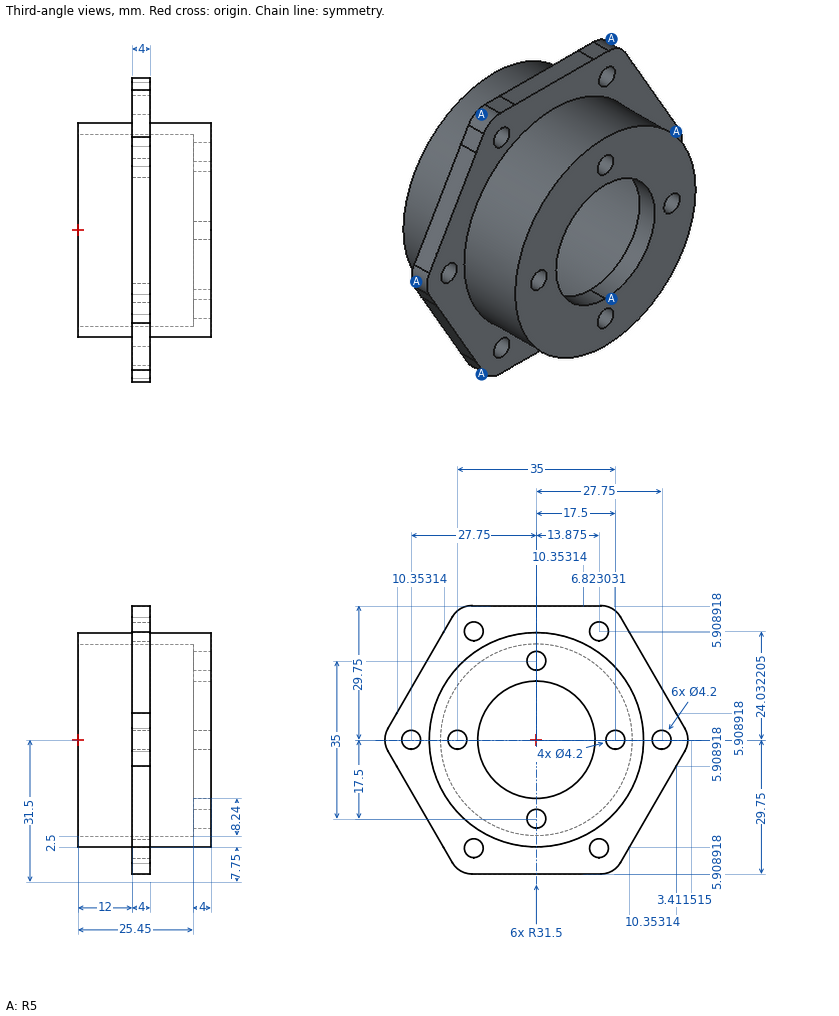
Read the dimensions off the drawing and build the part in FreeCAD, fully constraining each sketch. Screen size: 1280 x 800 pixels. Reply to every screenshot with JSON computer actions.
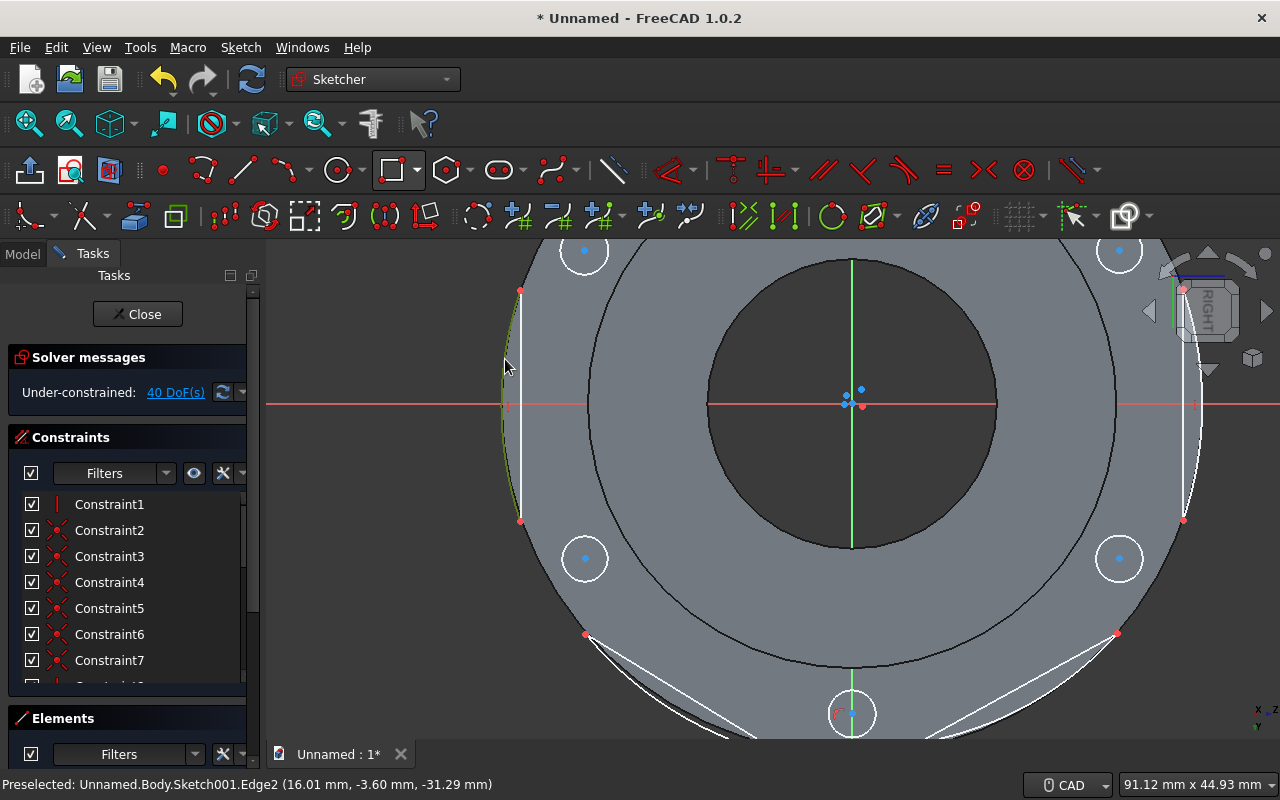
{"action": "scroll", "coordinate": [584, 558], "scroll_direction": "down", "scroll_amount": 4}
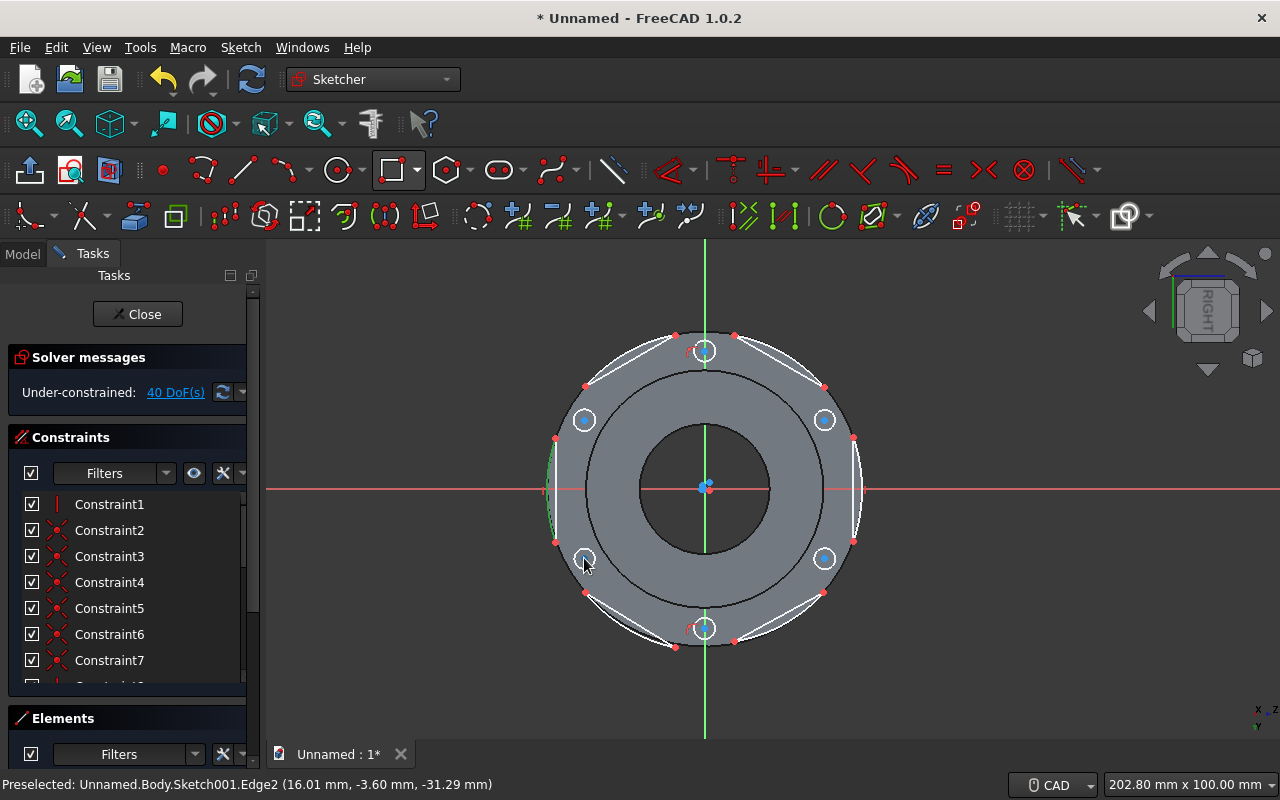
{"action": "scroll", "coordinate": [861, 511], "scroll_direction": "up", "scroll_amount": 4}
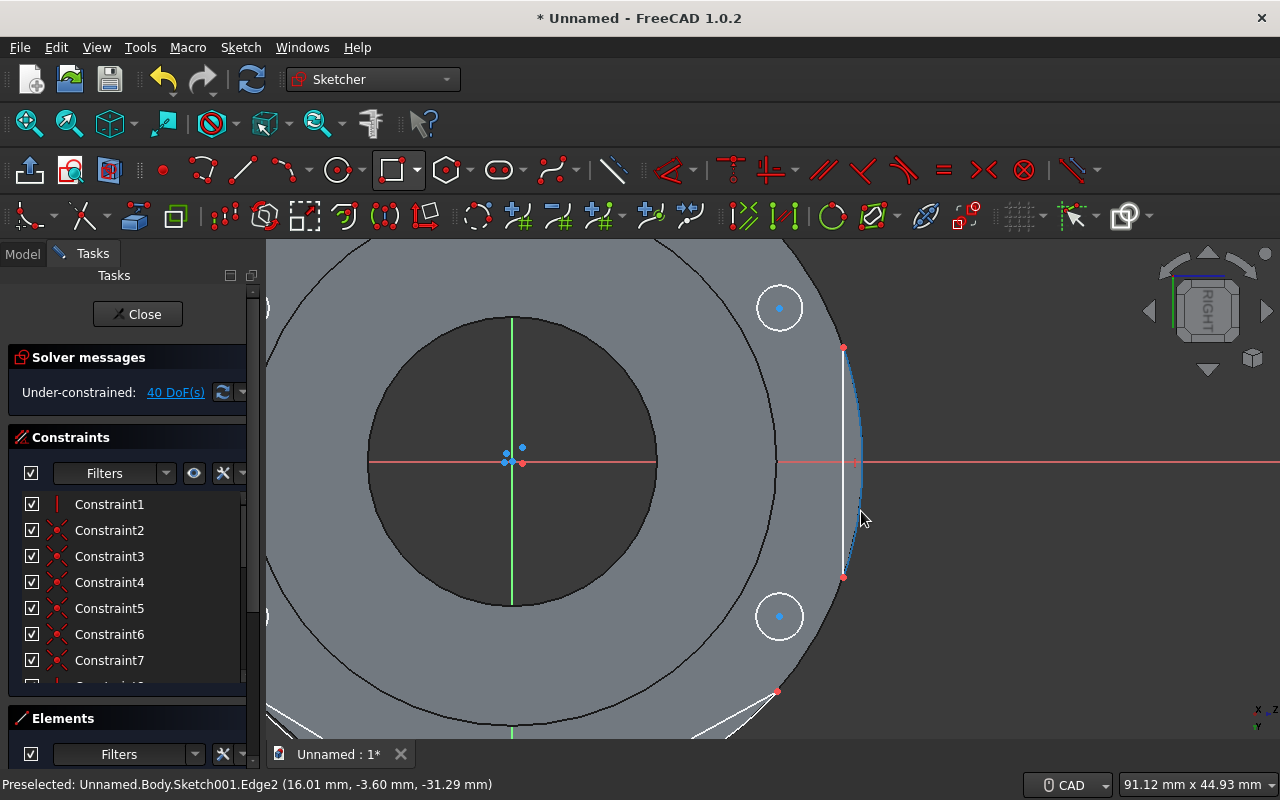
{"action": "left_click", "coordinate": [859, 509]}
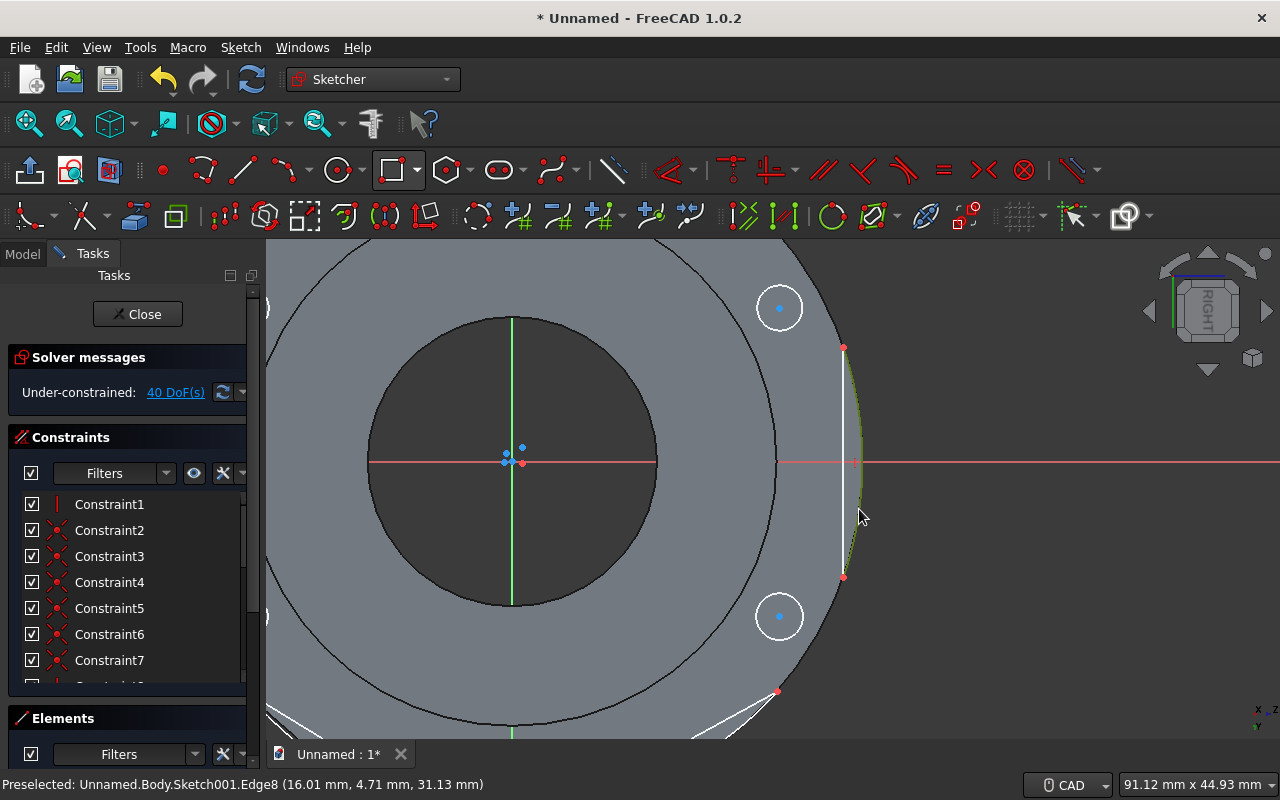
{"action": "left_click", "coordinate": [732, 170]}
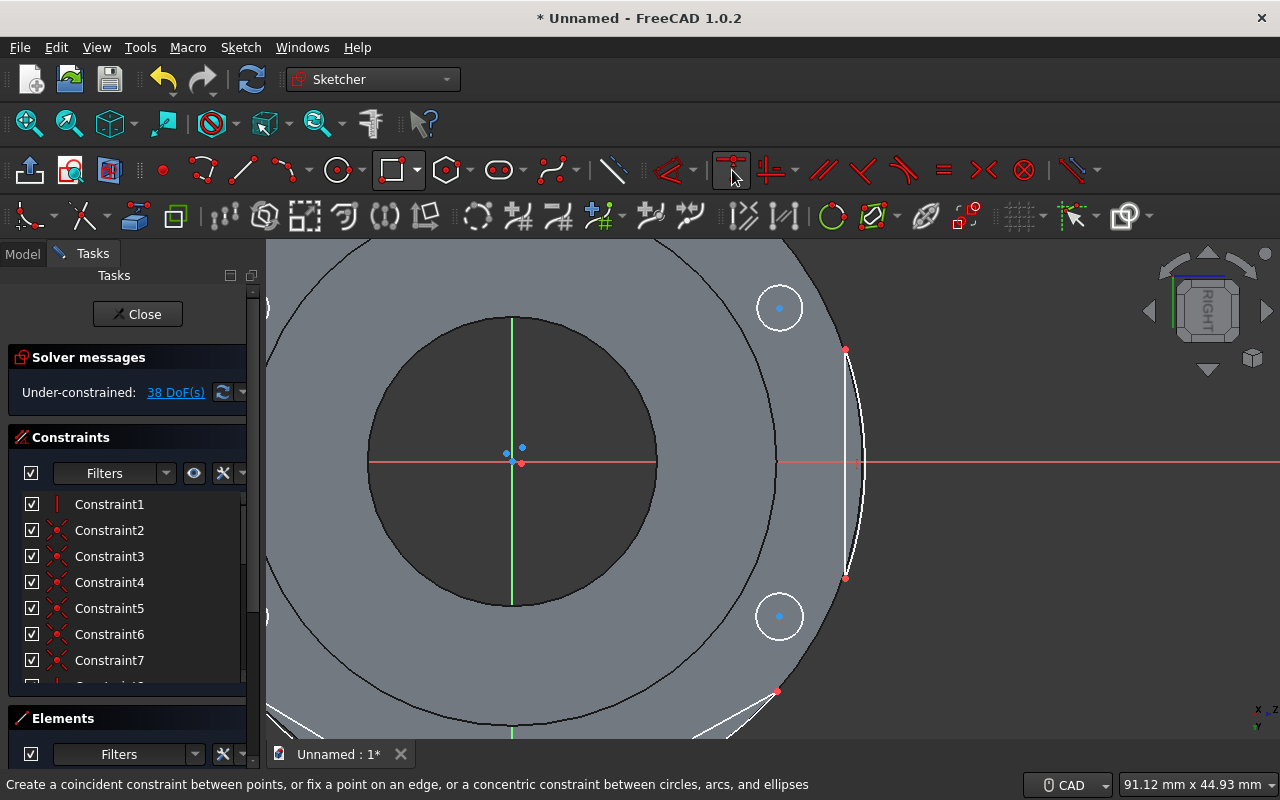
{"action": "scroll", "coordinate": [861, 511], "scroll_direction": "down", "scroll_amount": 4}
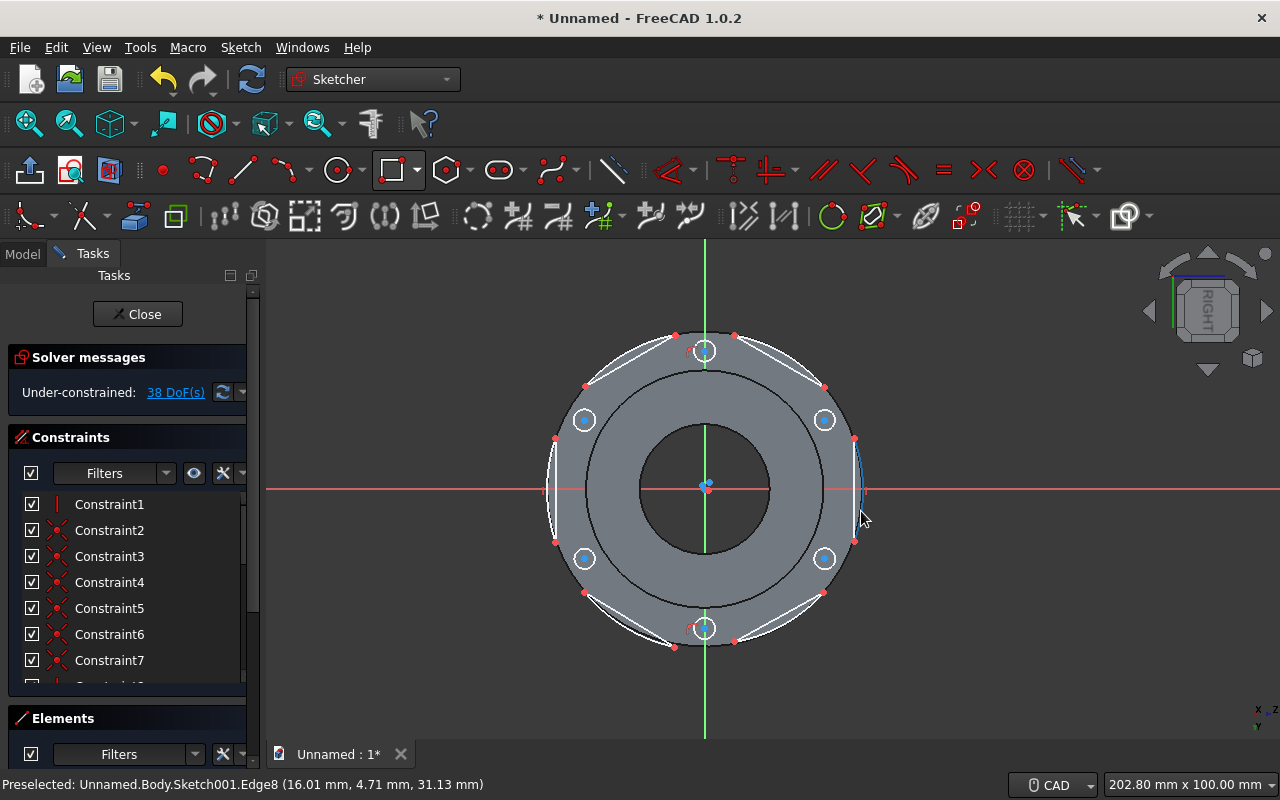
{"action": "scroll", "coordinate": [548, 469], "scroll_direction": "up", "scroll_amount": 4}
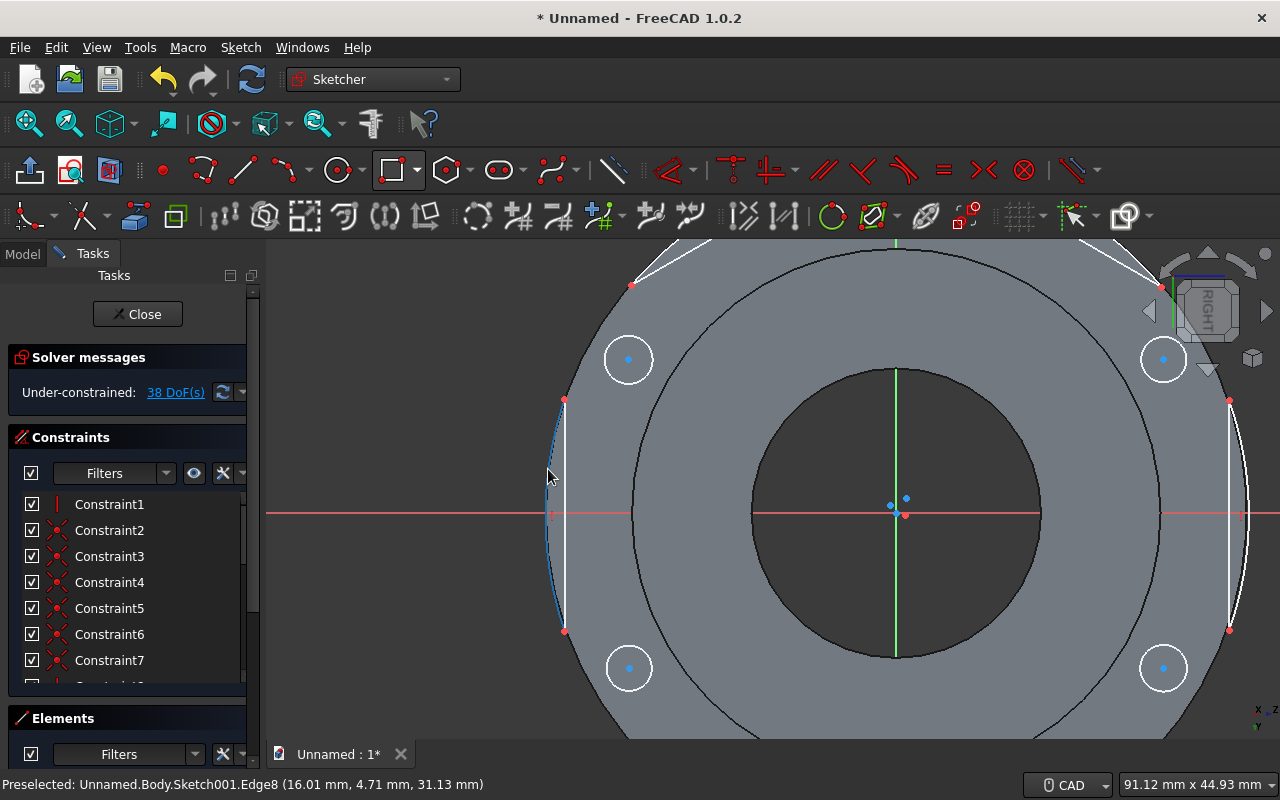
{"action": "left_click", "coordinate": [549, 468]}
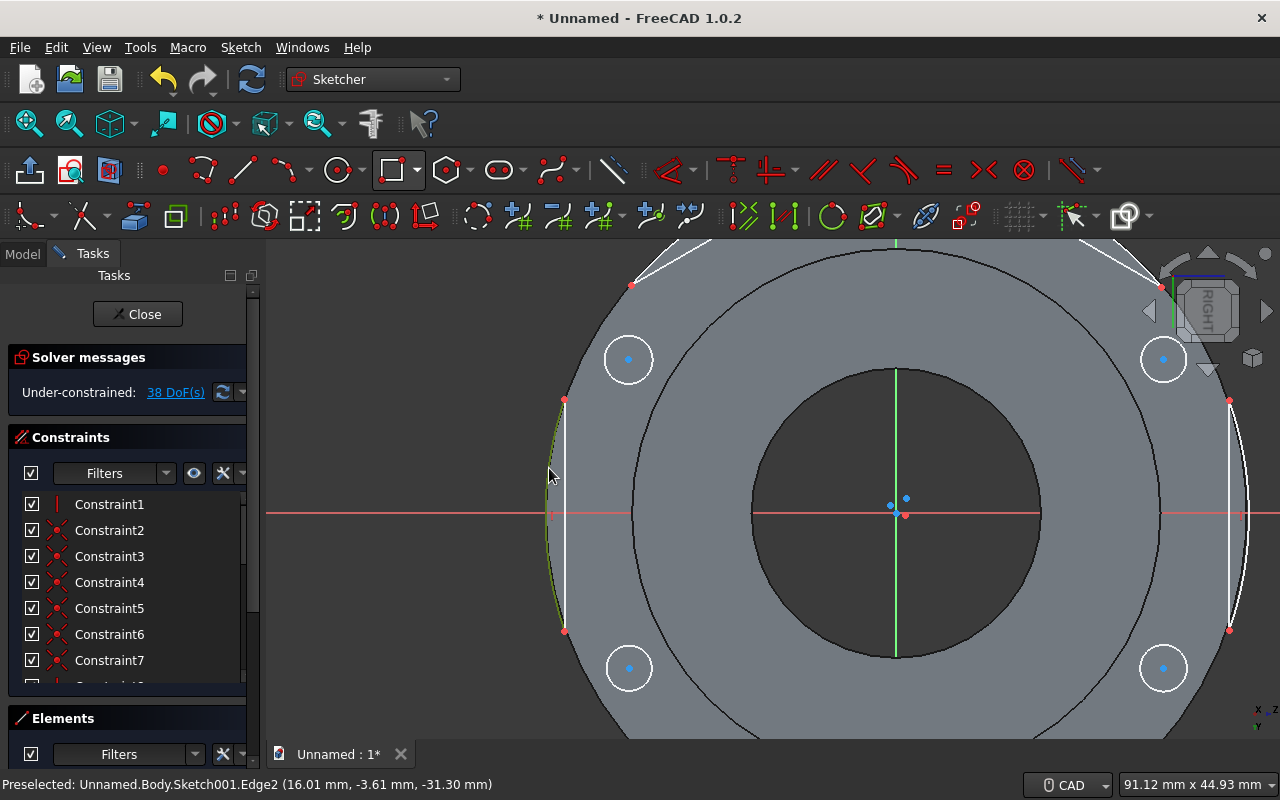
{"action": "scroll", "coordinate": [548, 469], "scroll_direction": "down", "scroll_amount": 4}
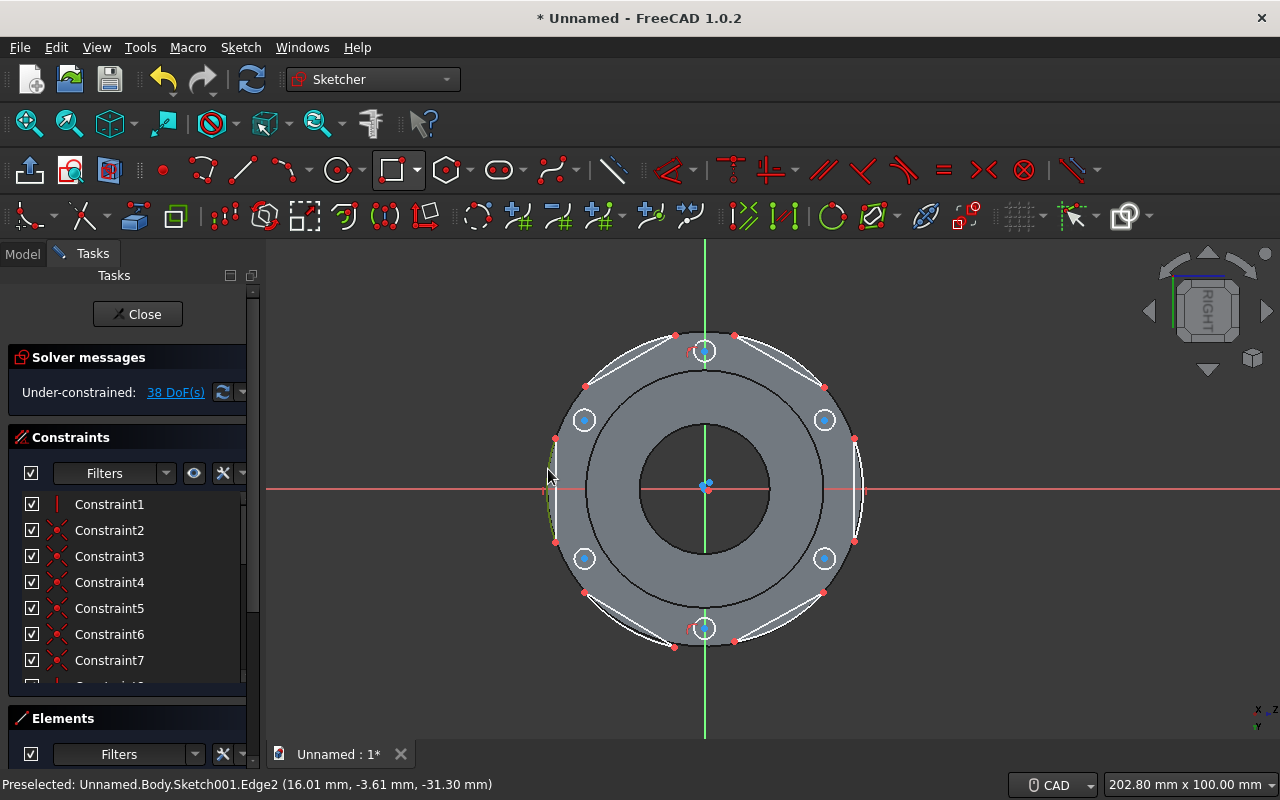
{"action": "scroll", "coordinate": [801, 365], "scroll_direction": "up", "scroll_amount": 3}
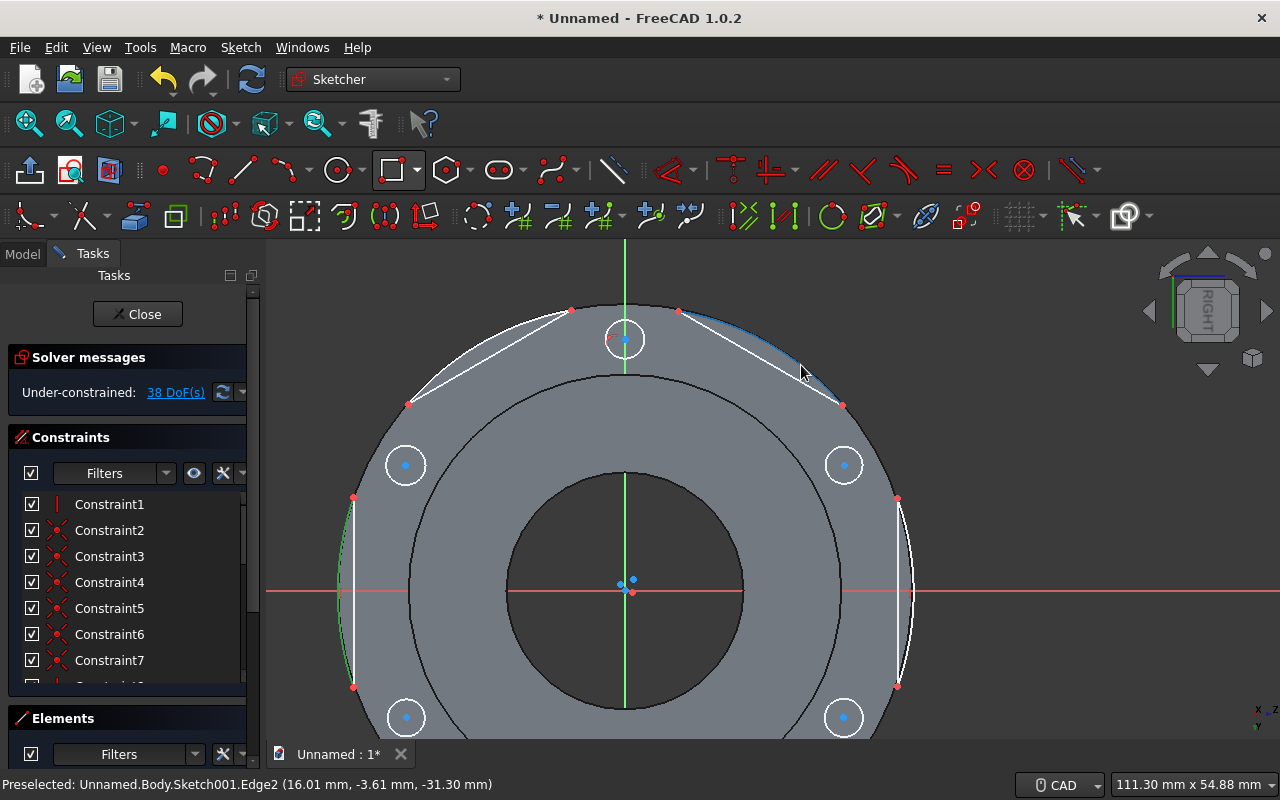
{"action": "left_click", "coordinate": [801, 365]}